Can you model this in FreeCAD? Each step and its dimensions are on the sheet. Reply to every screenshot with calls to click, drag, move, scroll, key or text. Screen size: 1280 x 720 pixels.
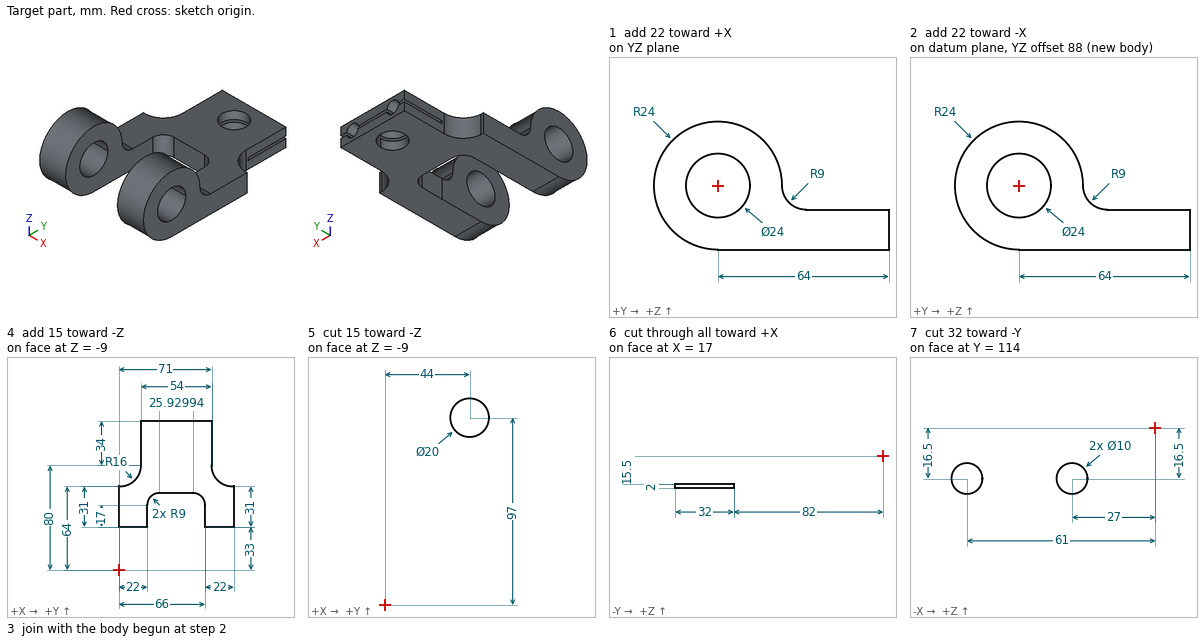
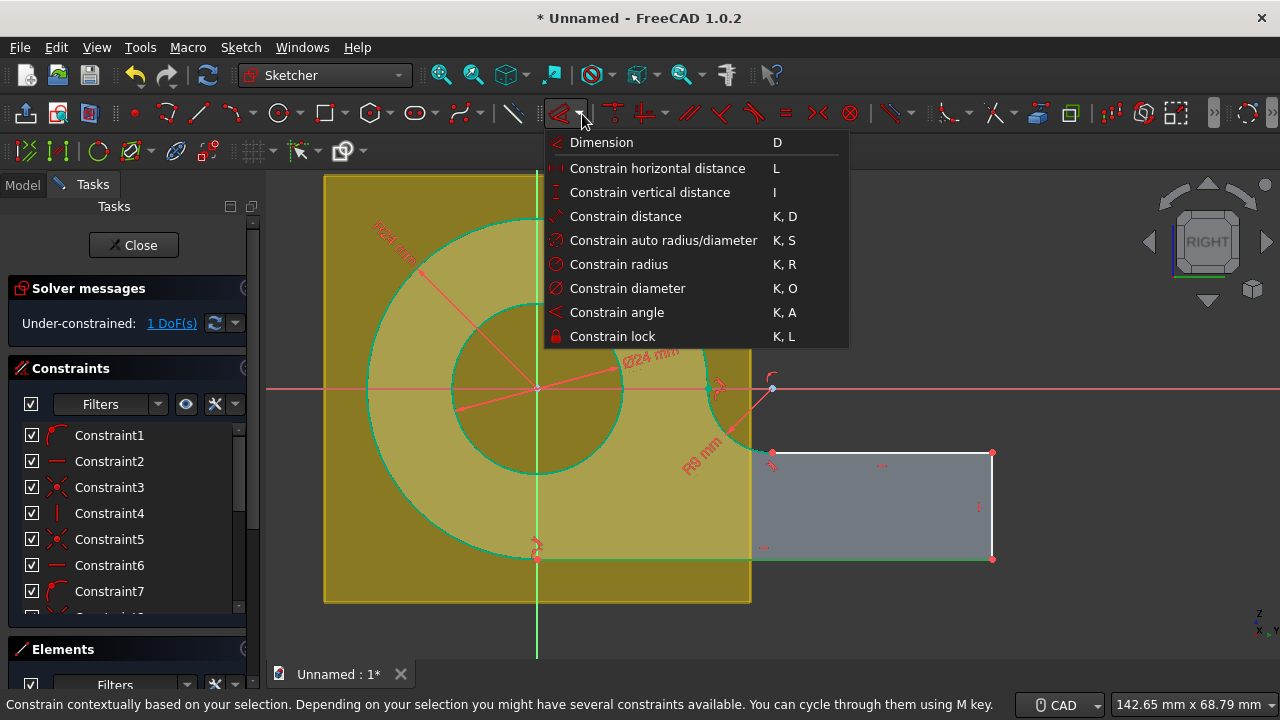
click(697, 168)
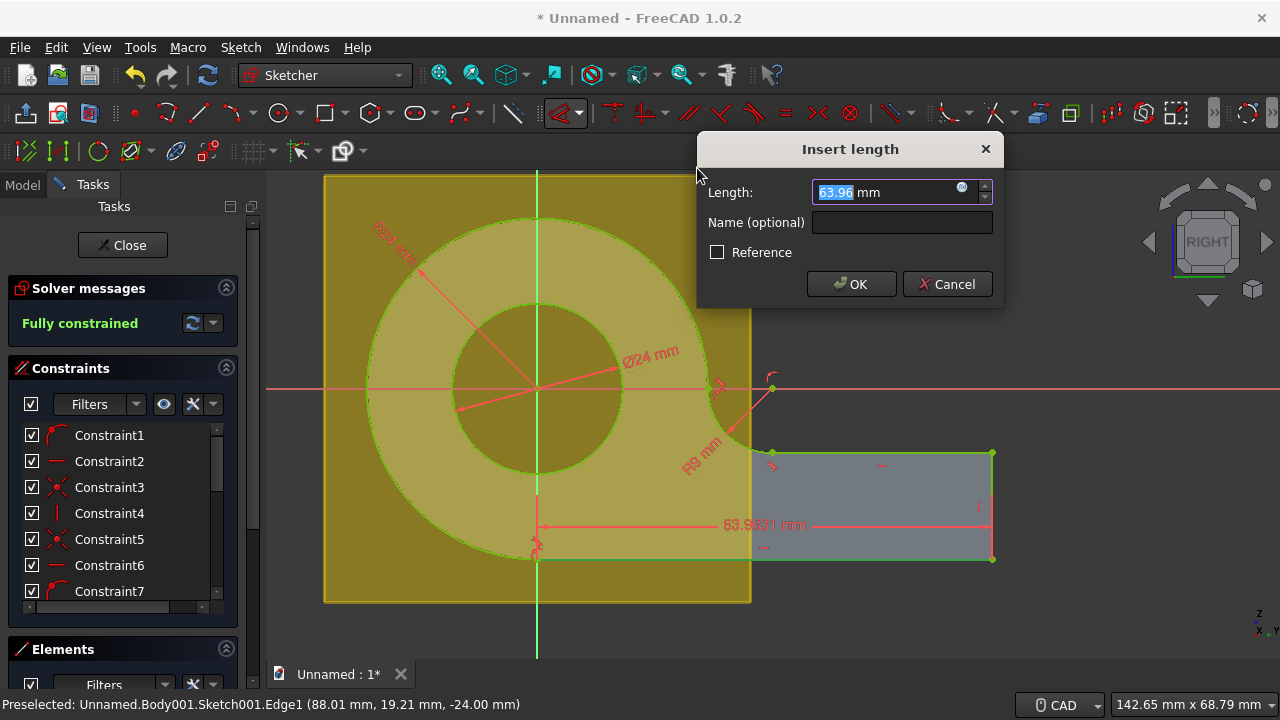
text(64)
key(Return)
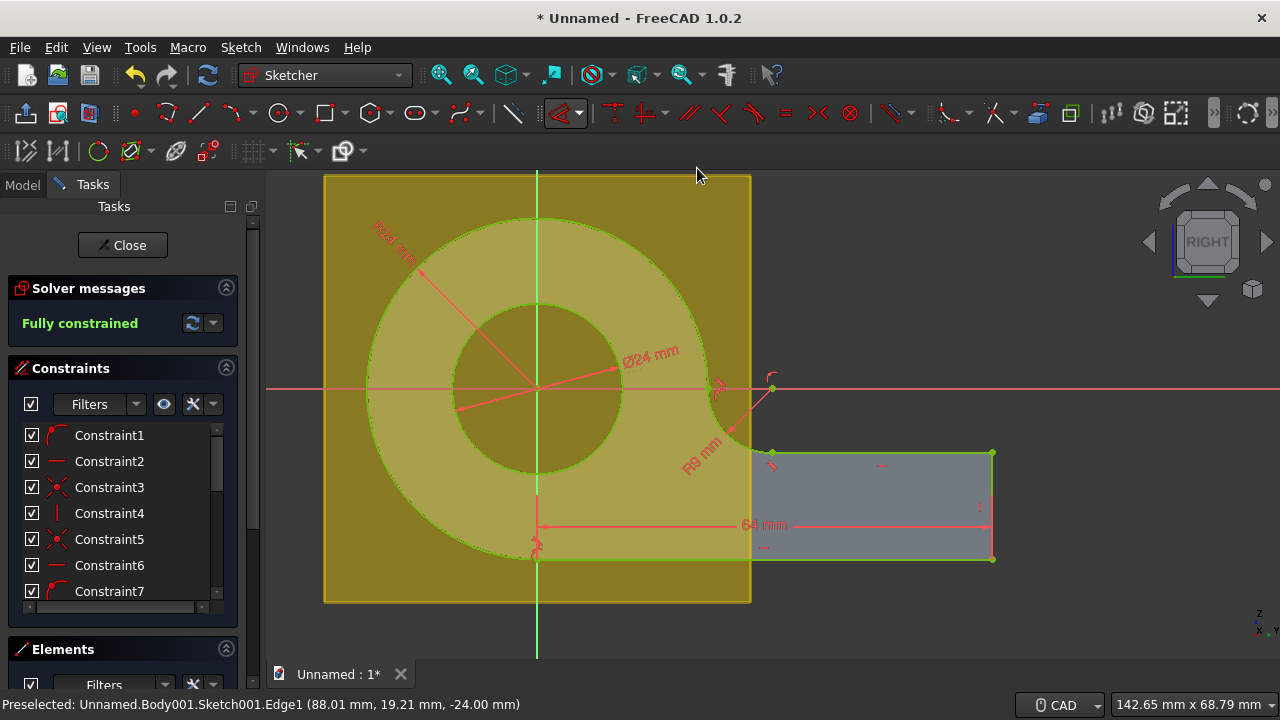
click(123, 245)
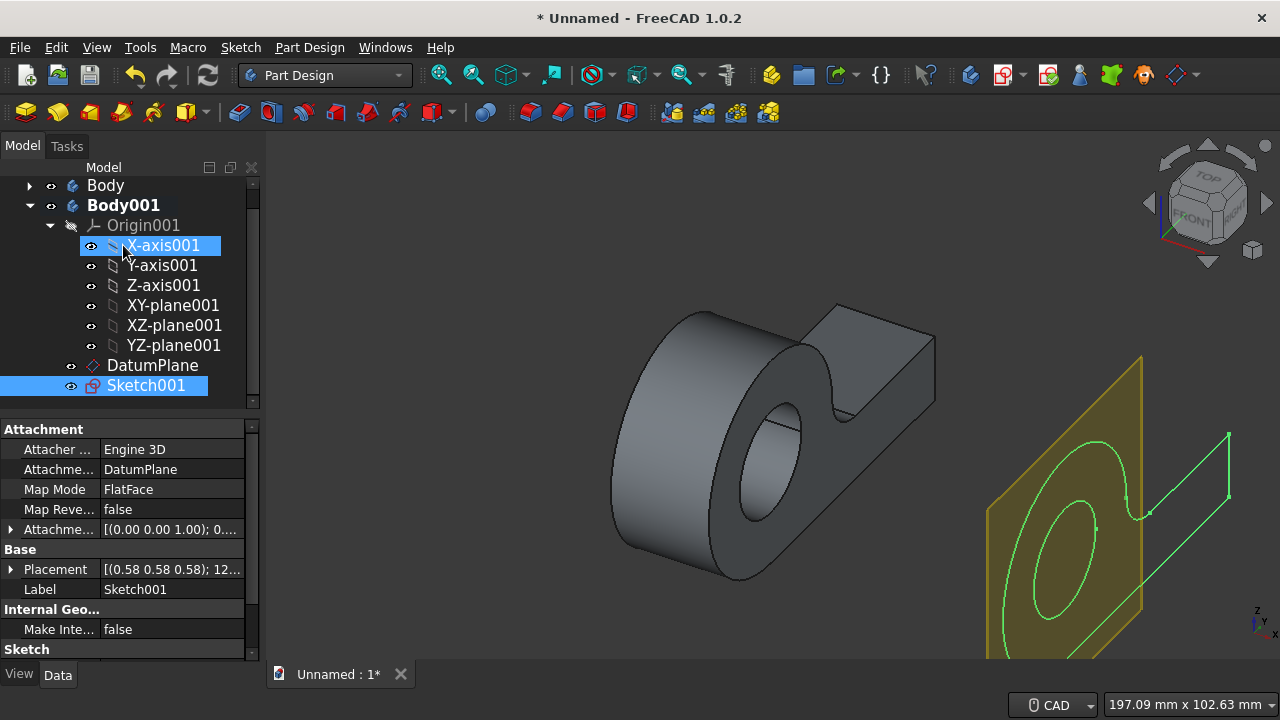
click(26, 112)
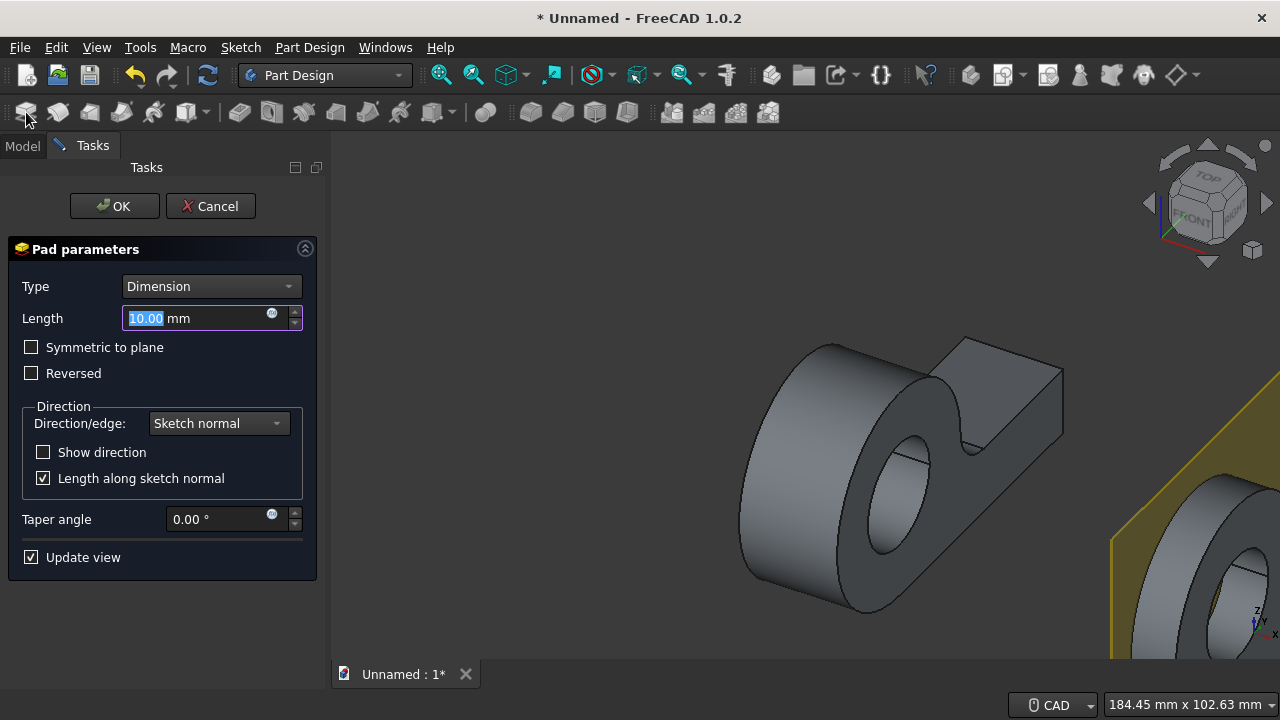
text(22)
key(Tab)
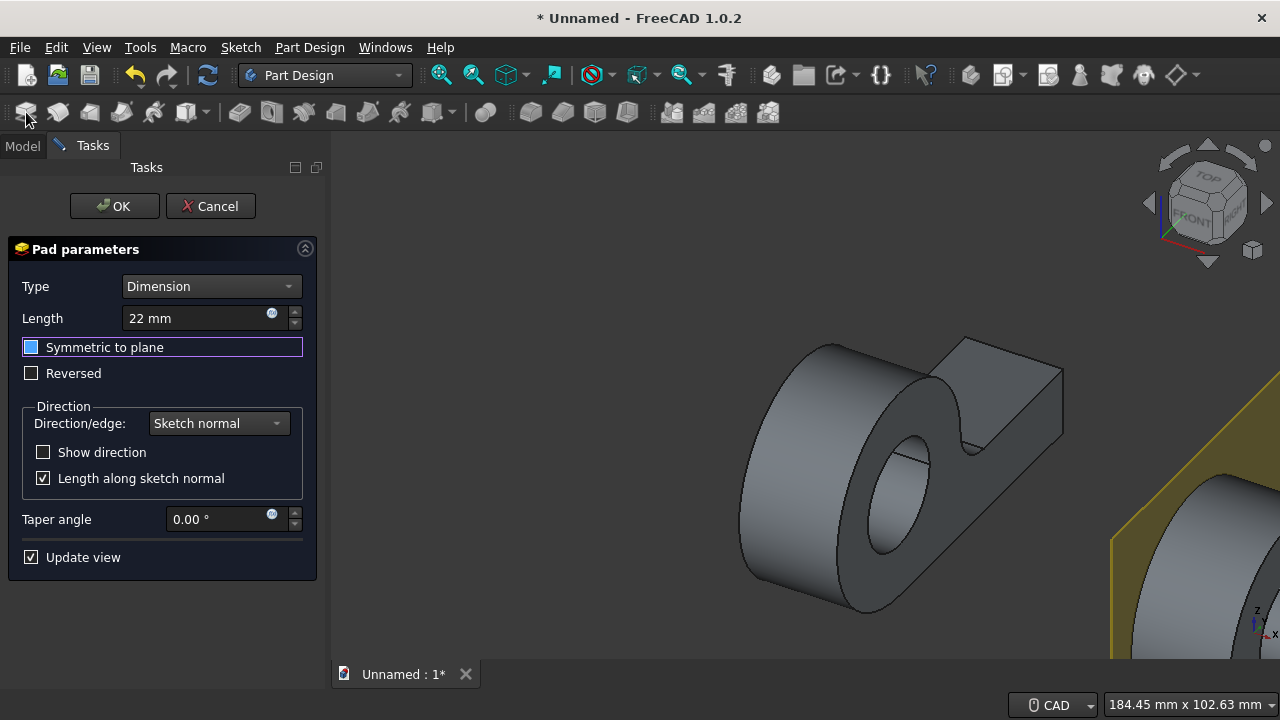
click(30, 373)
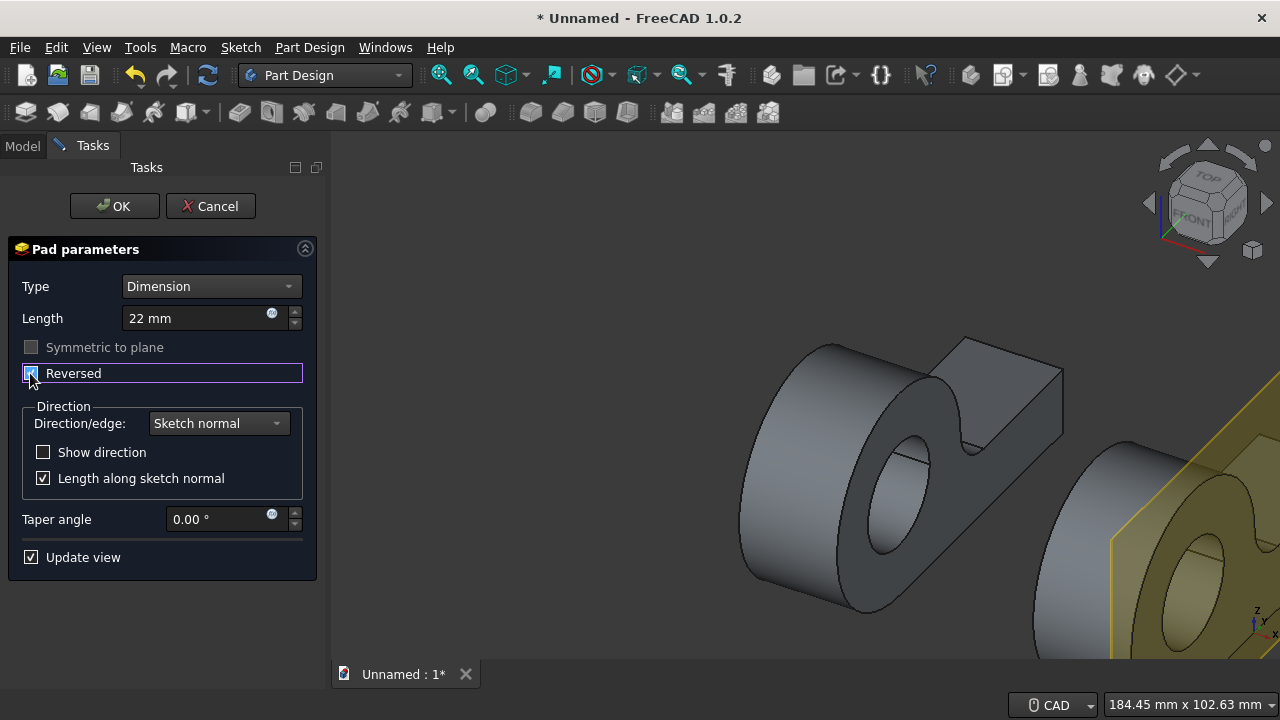
click(115, 206)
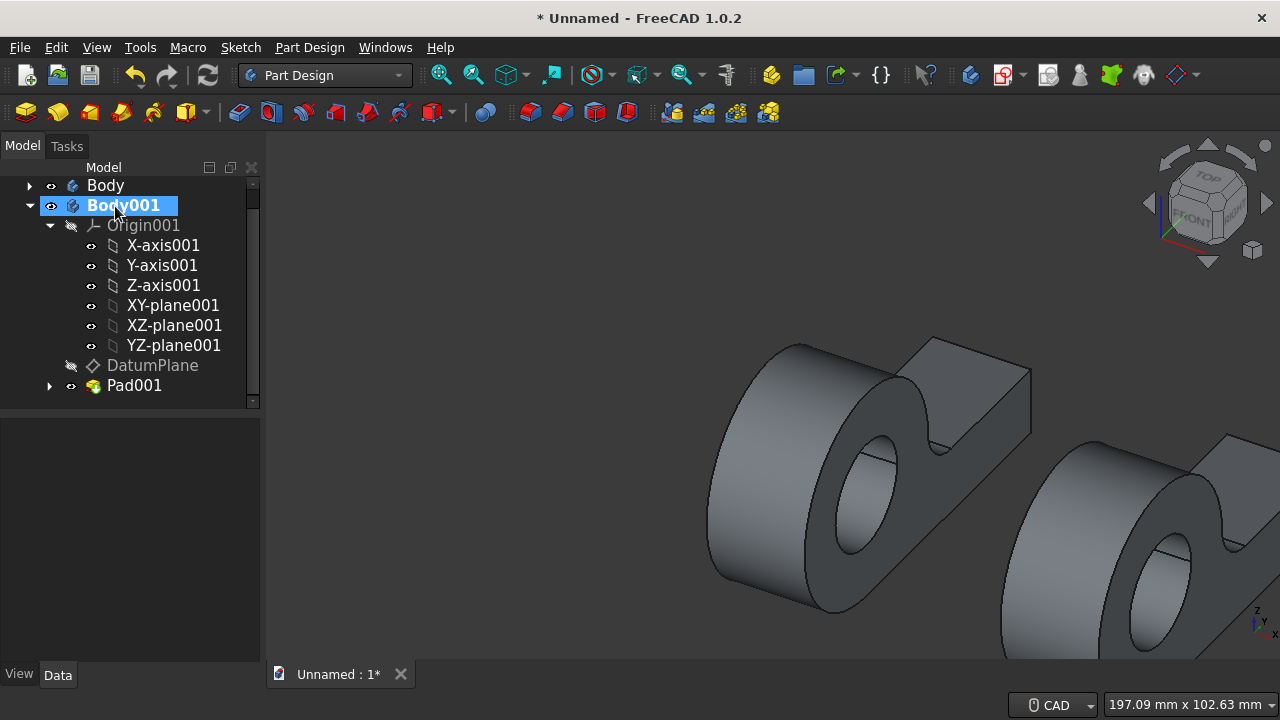
click(442, 76)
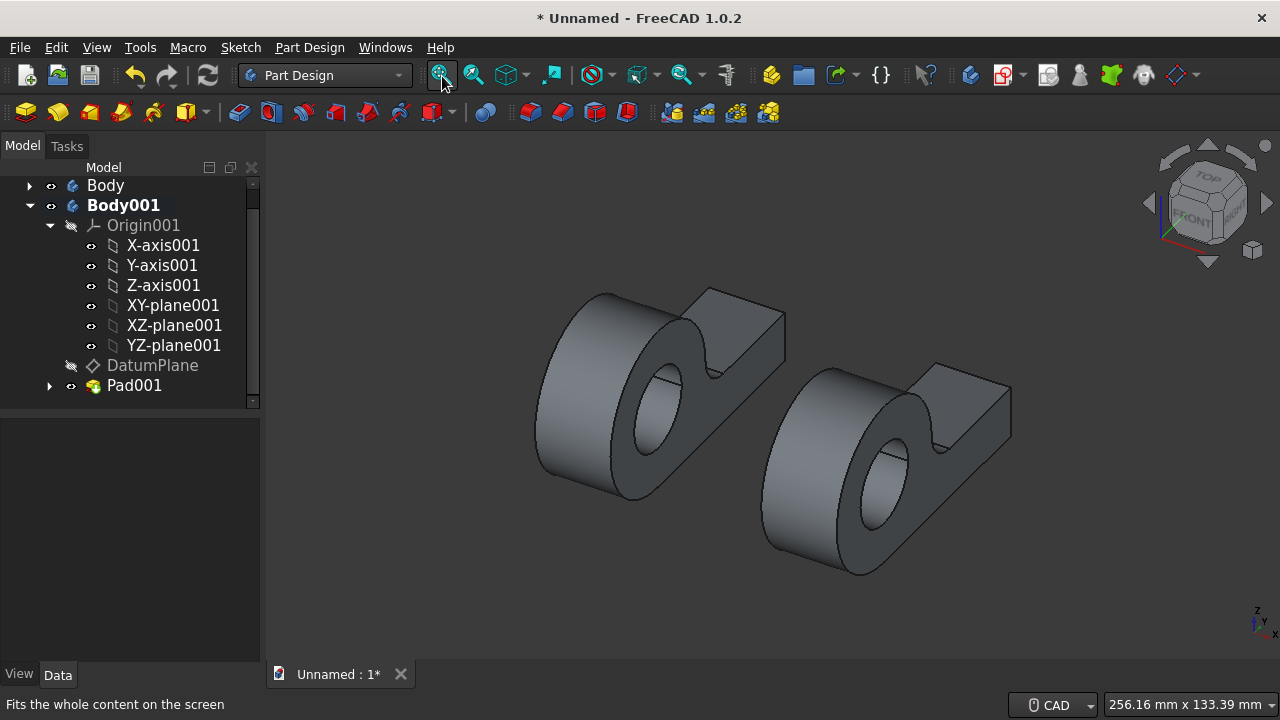
double_click(96, 186)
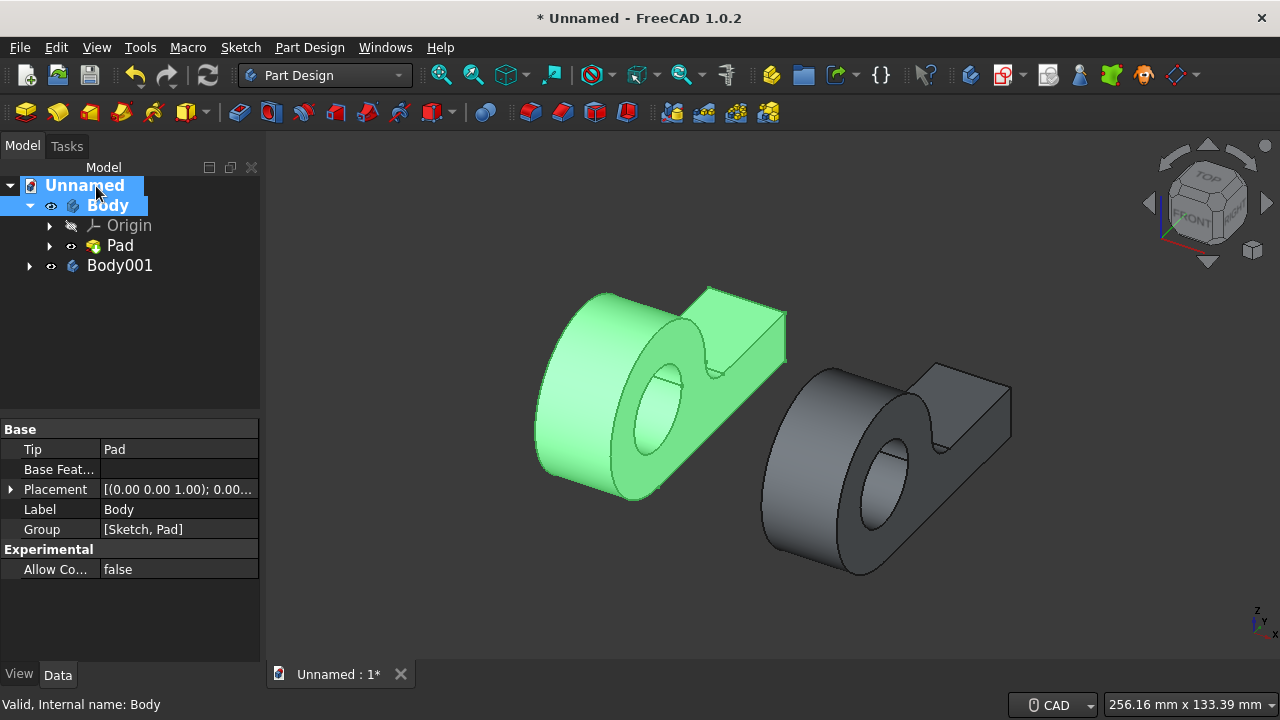
click(96, 206)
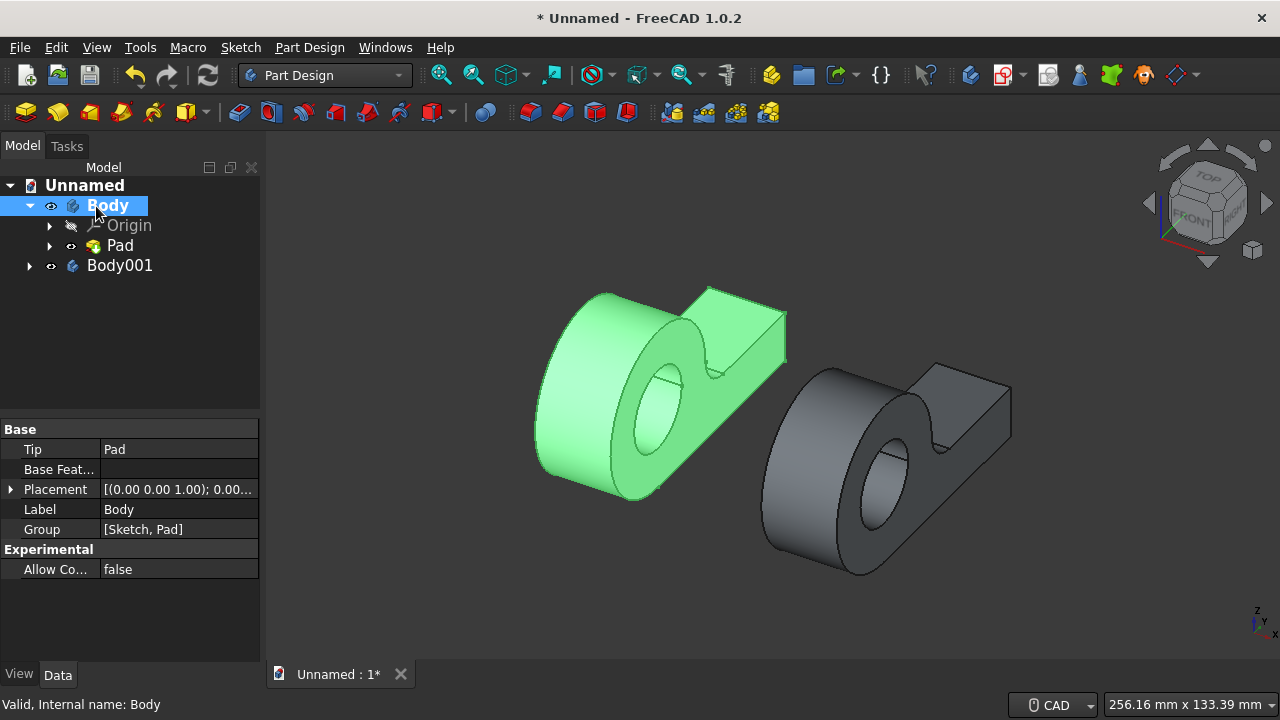
click(146, 569)